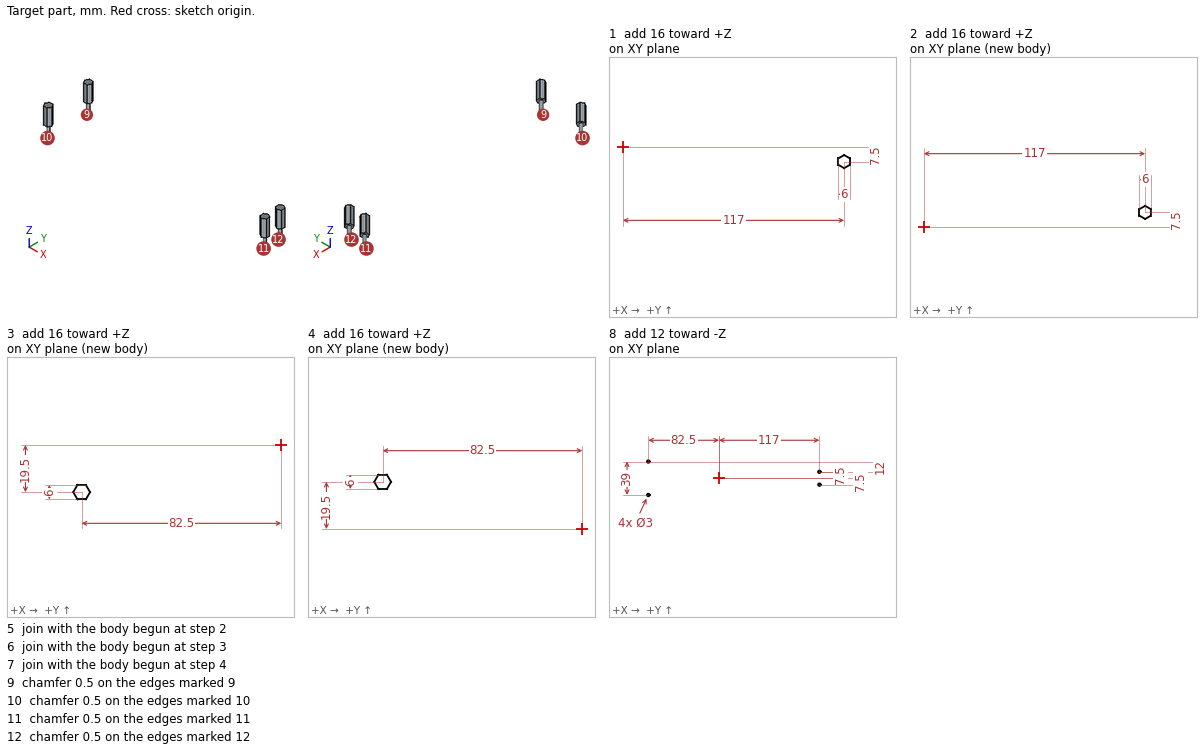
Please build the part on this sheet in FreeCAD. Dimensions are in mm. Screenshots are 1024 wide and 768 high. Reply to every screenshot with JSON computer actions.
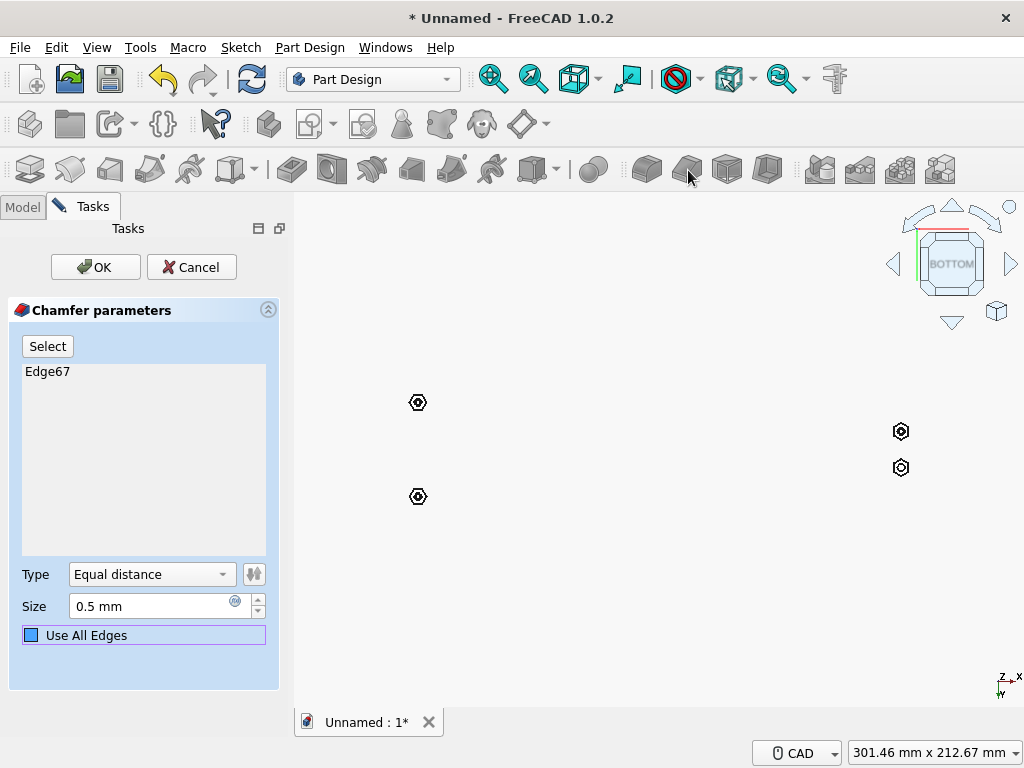
{"action": "left_click", "coordinate": [96, 267]}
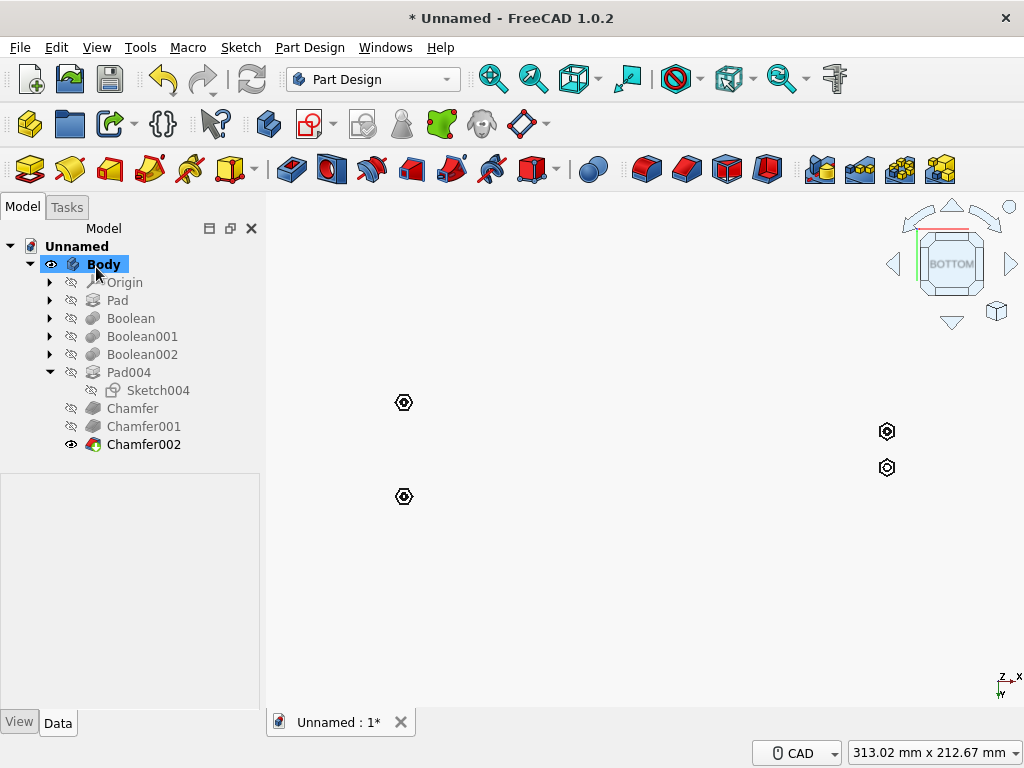
{"action": "left_click", "coordinate": [883, 467]}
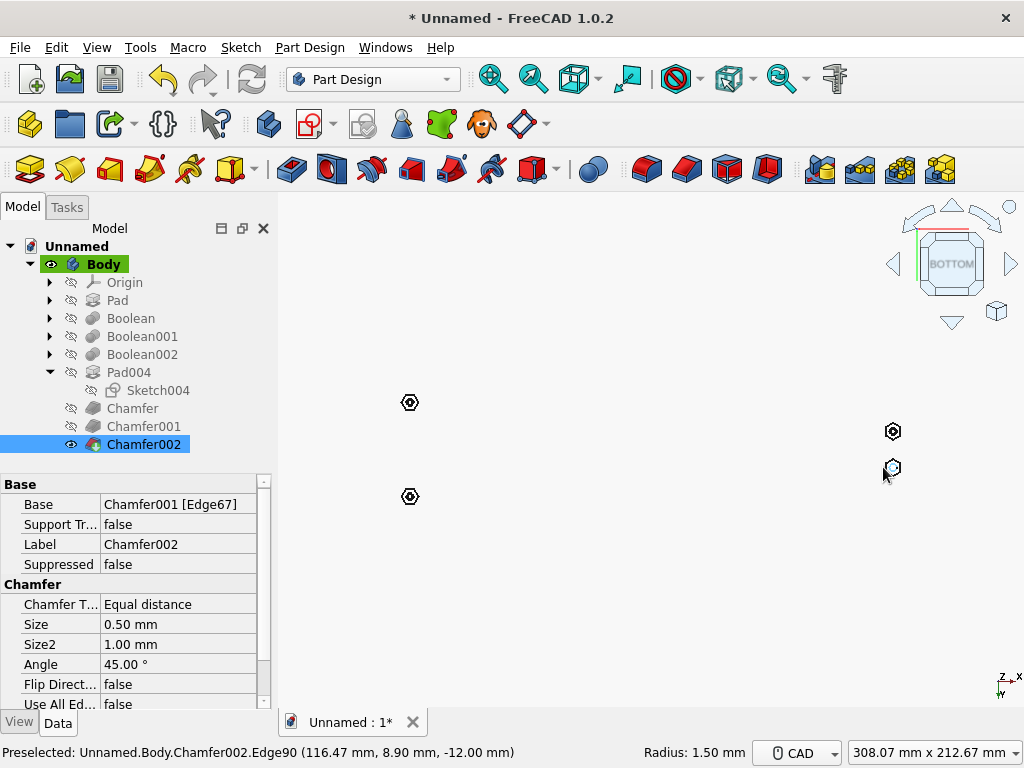
{"action": "left_click", "coordinate": [688, 170]}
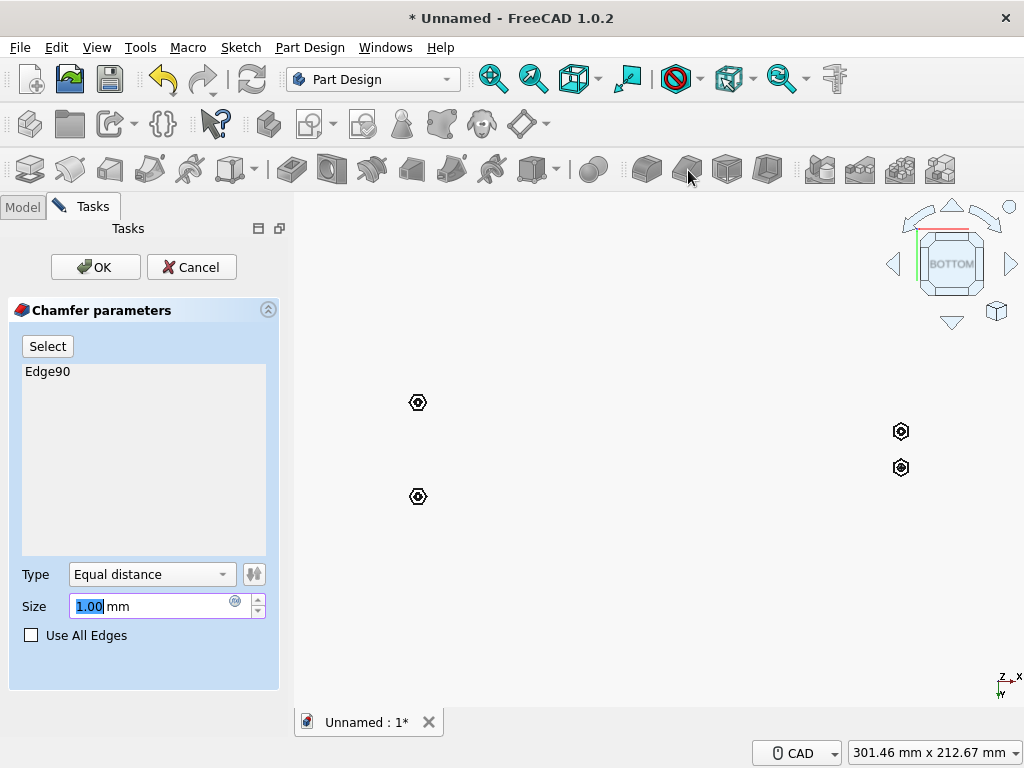
{"action": "type", "text": "0.5"}
{"action": "key", "text": "Tab"}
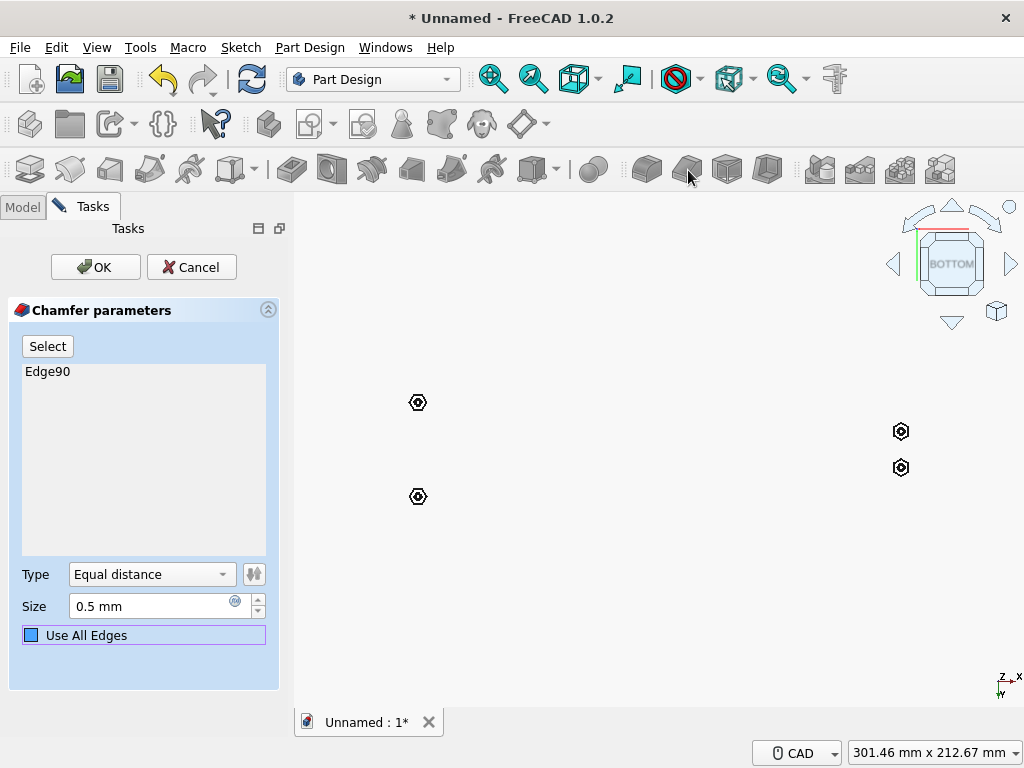
{"action": "left_click", "coordinate": [96, 267]}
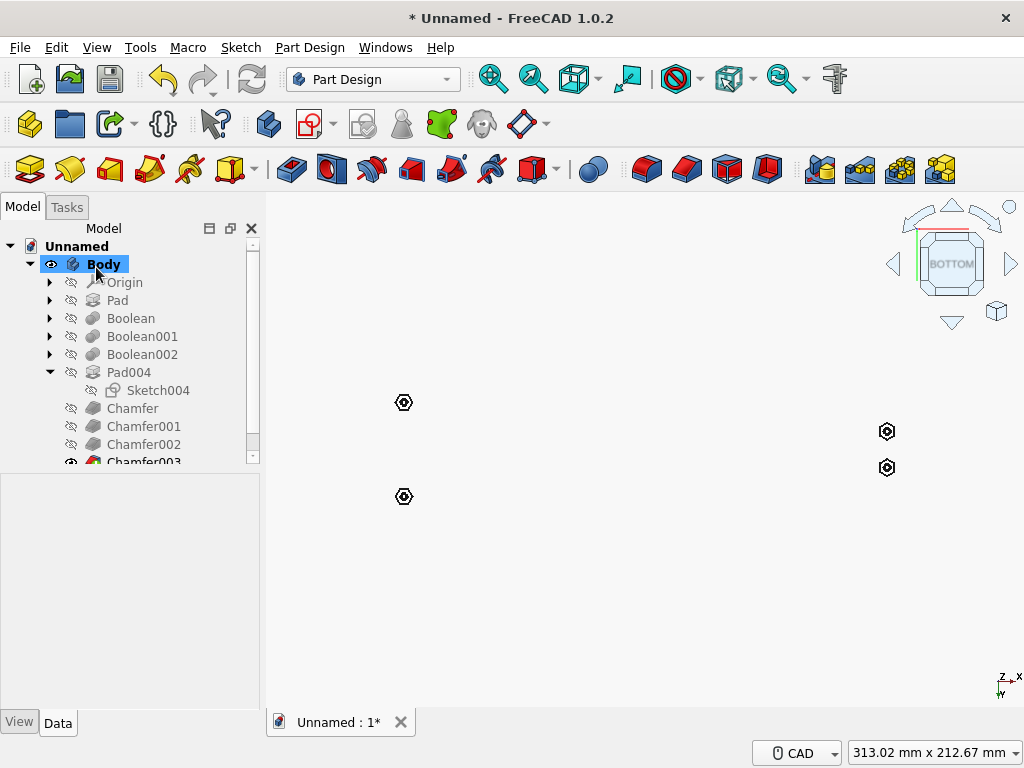
{"action": "key", "text": "0"}